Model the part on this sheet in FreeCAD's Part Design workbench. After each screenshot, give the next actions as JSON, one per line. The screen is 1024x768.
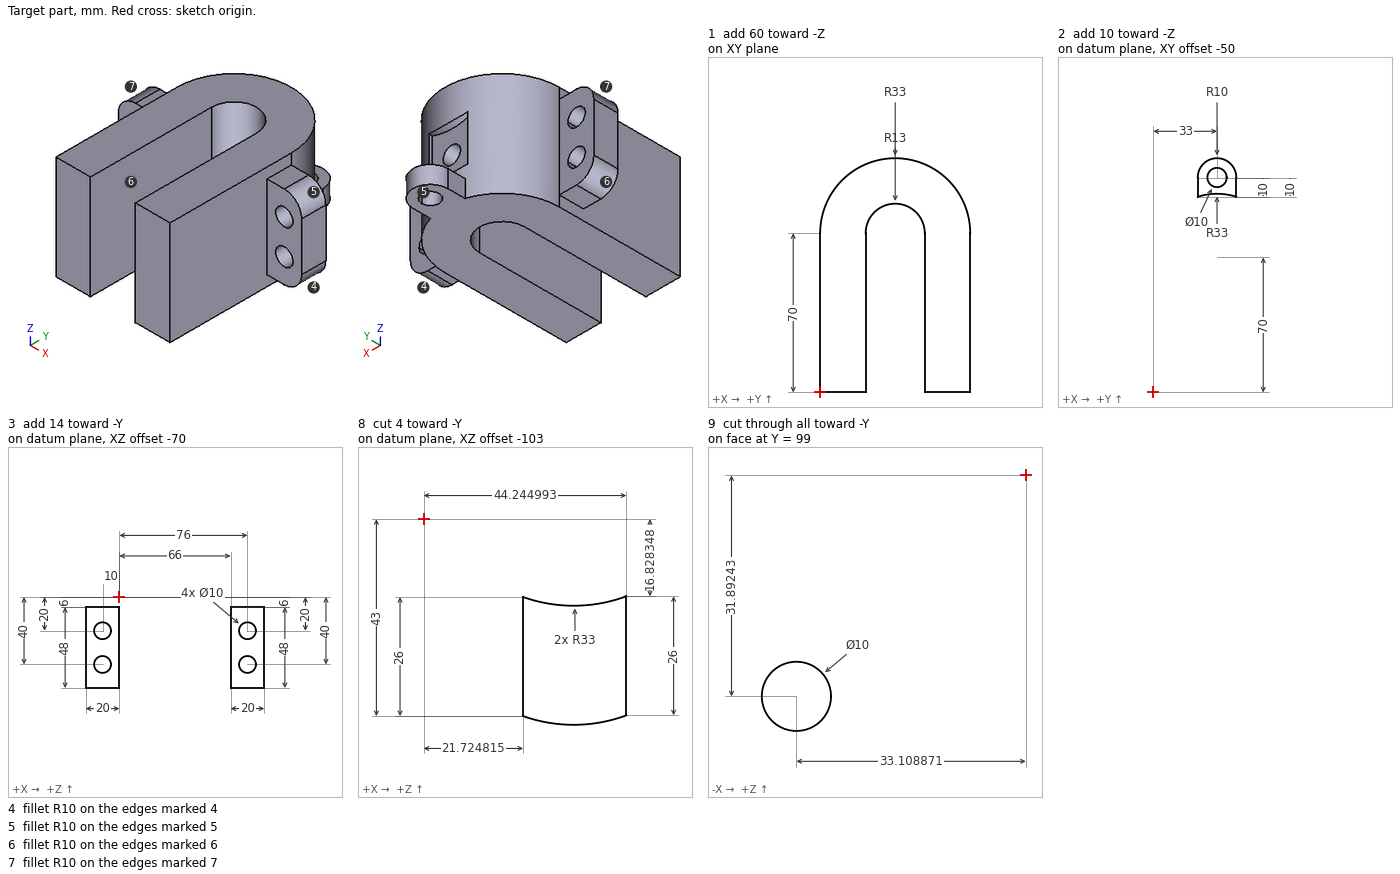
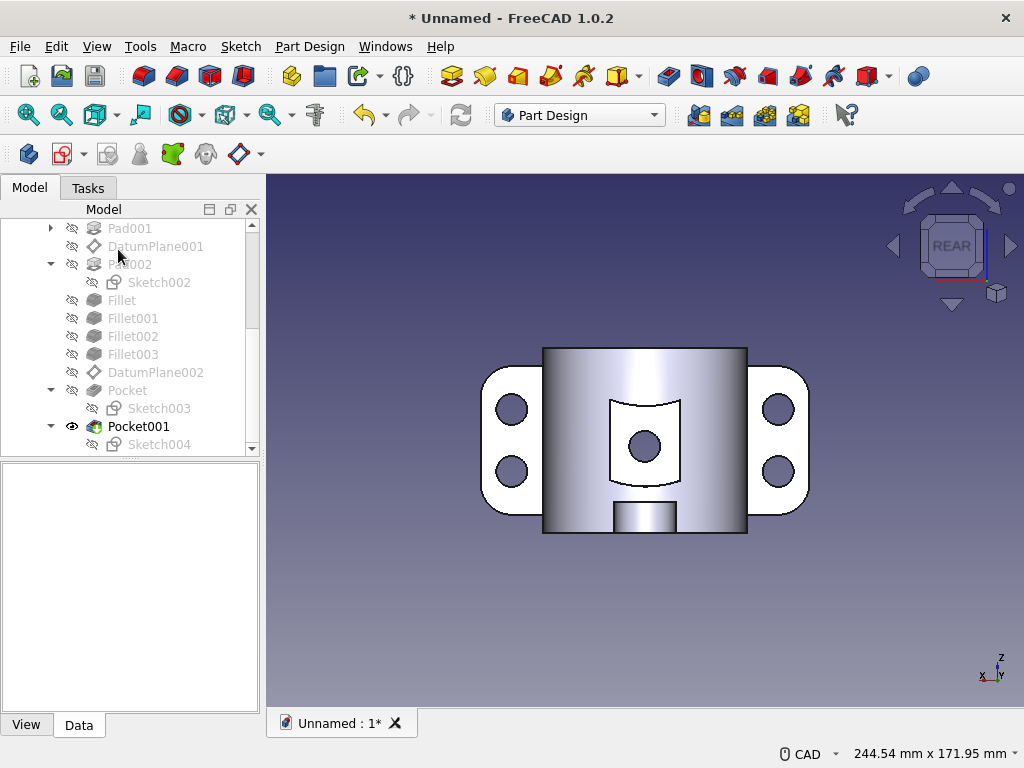
{"action": "key", "text": "0"}